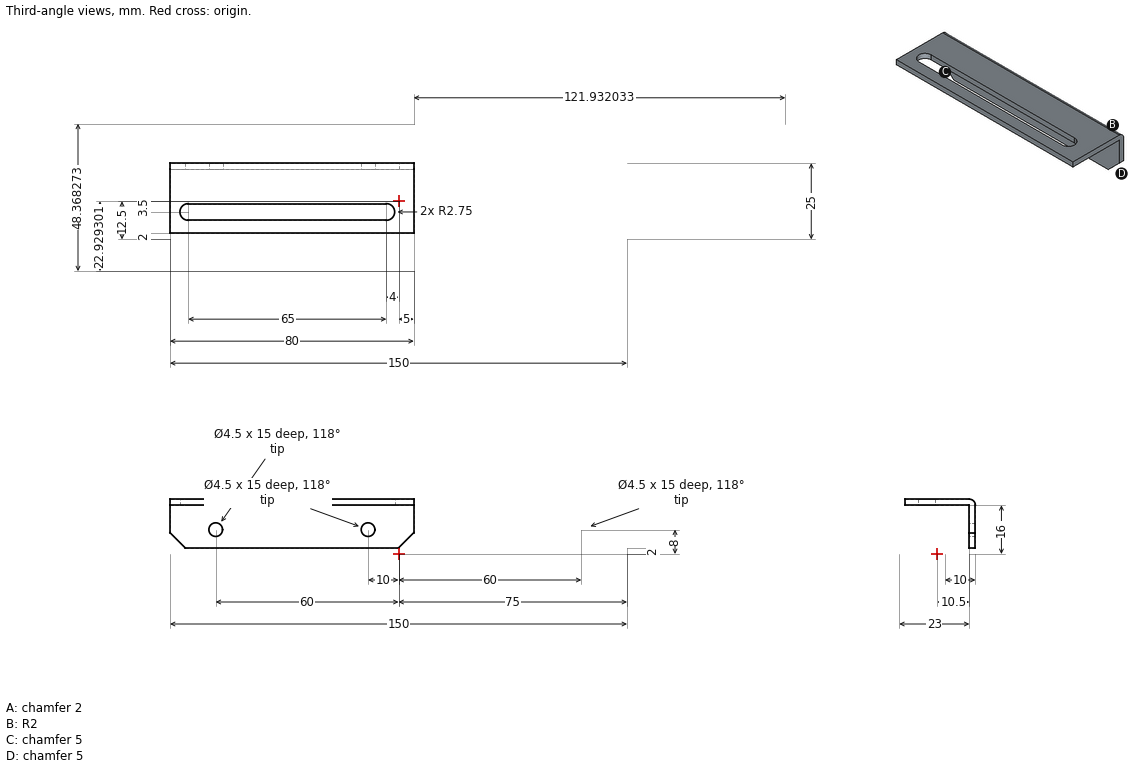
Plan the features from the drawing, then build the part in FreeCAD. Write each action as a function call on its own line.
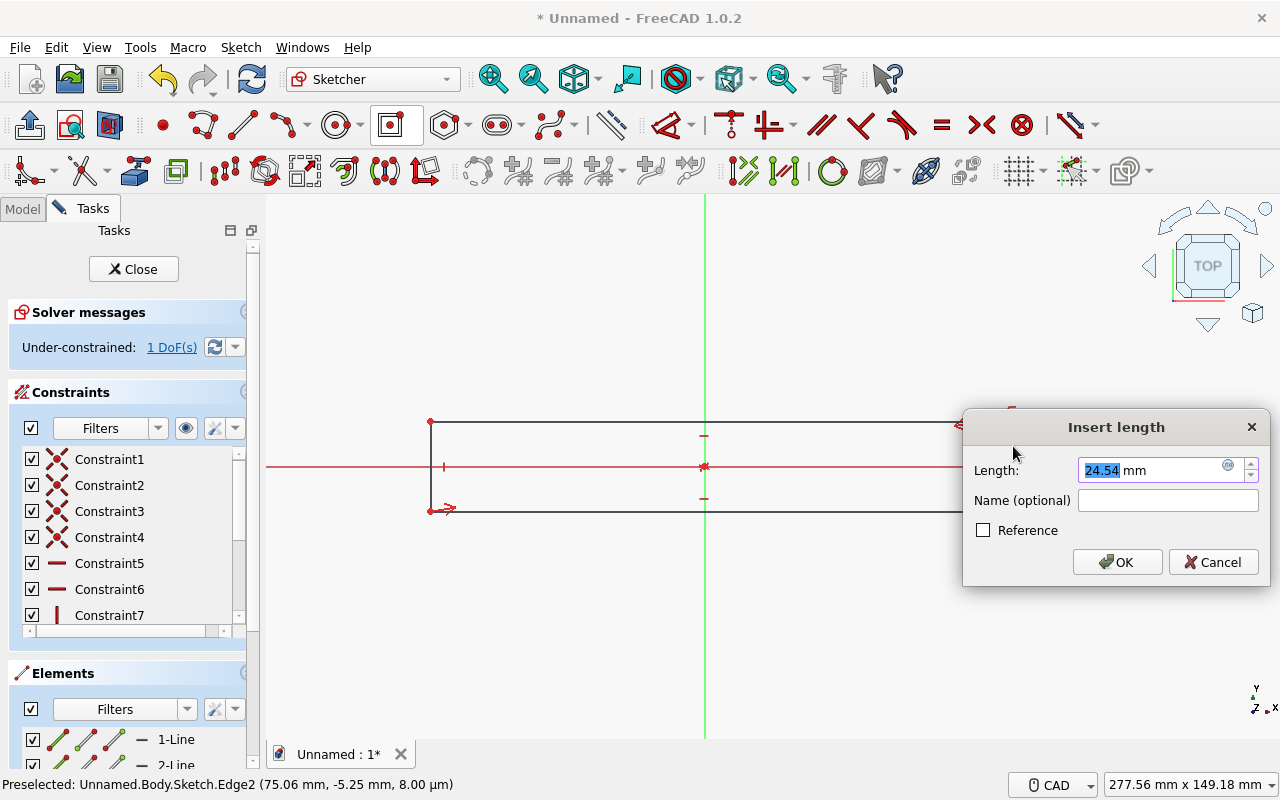
text(25)
key(Return)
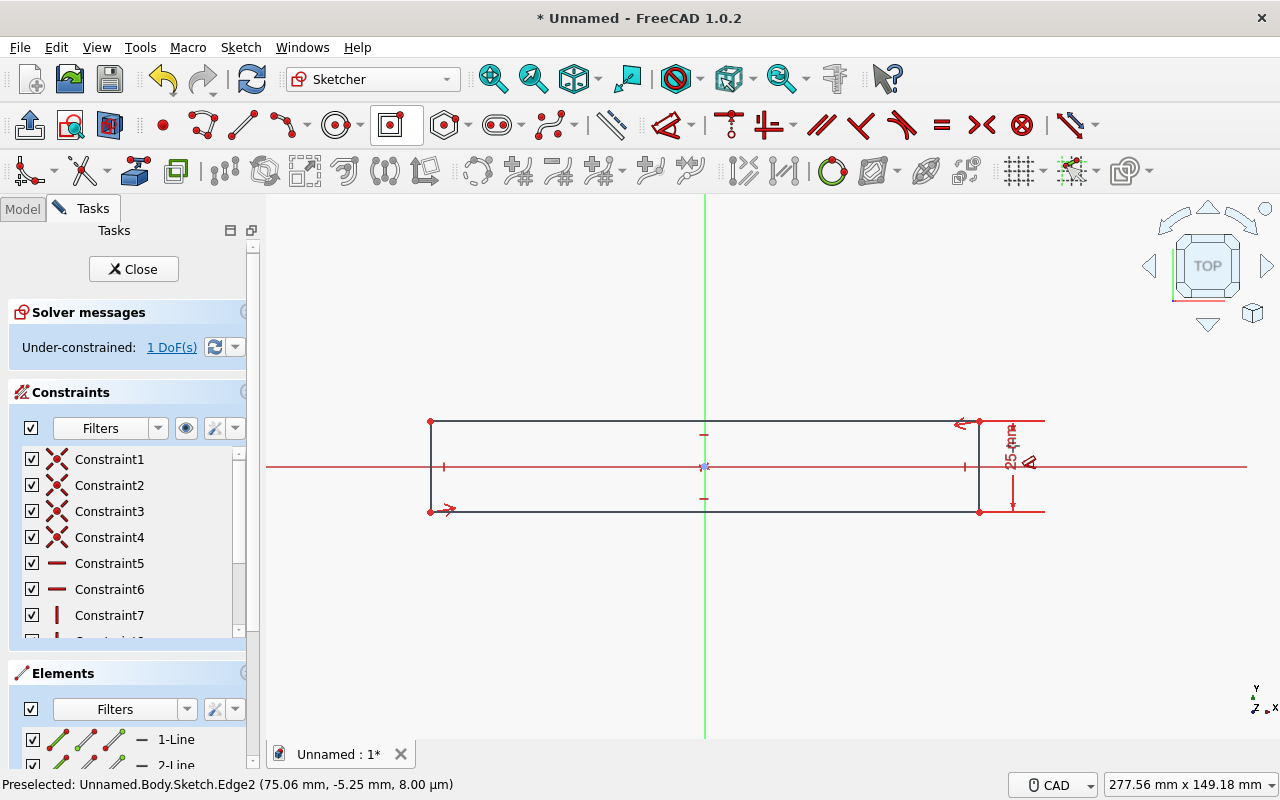
click(595, 512)
click(579, 546)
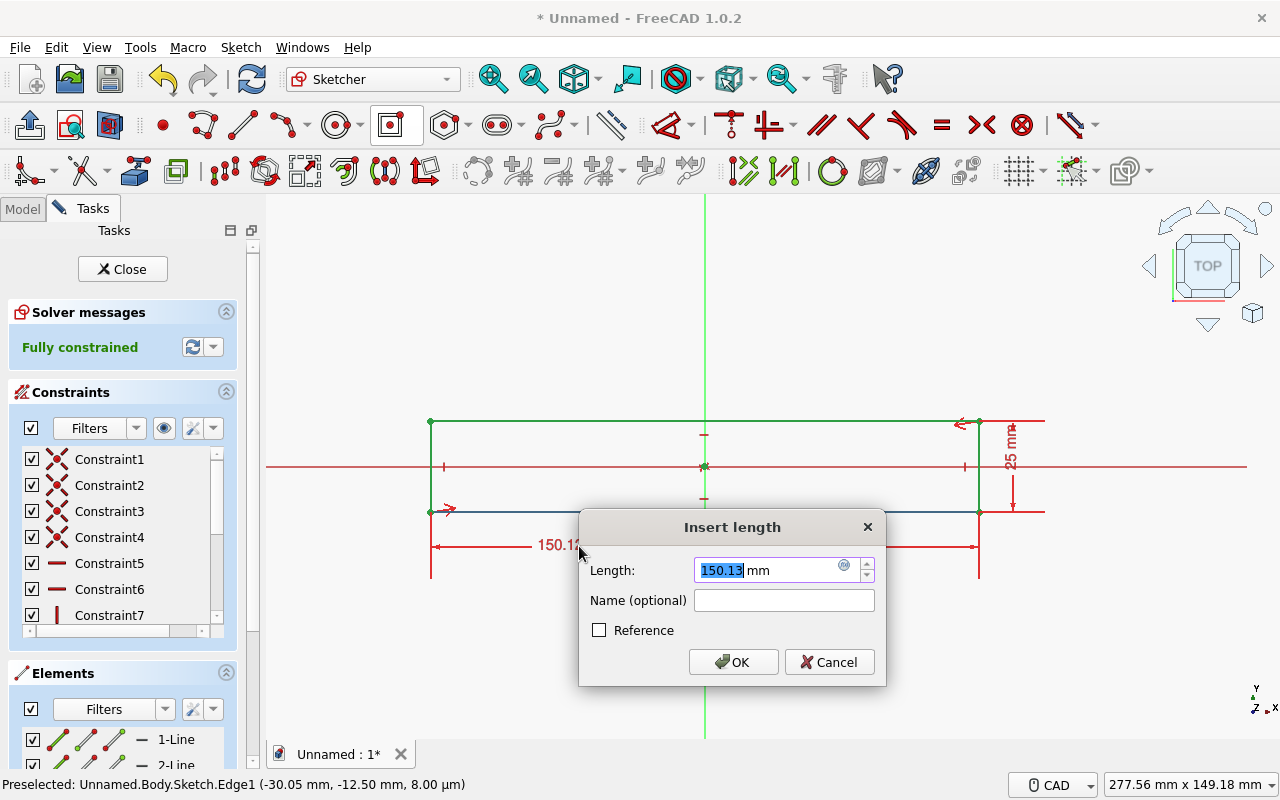
text(150)
key(Return)
key(Escape)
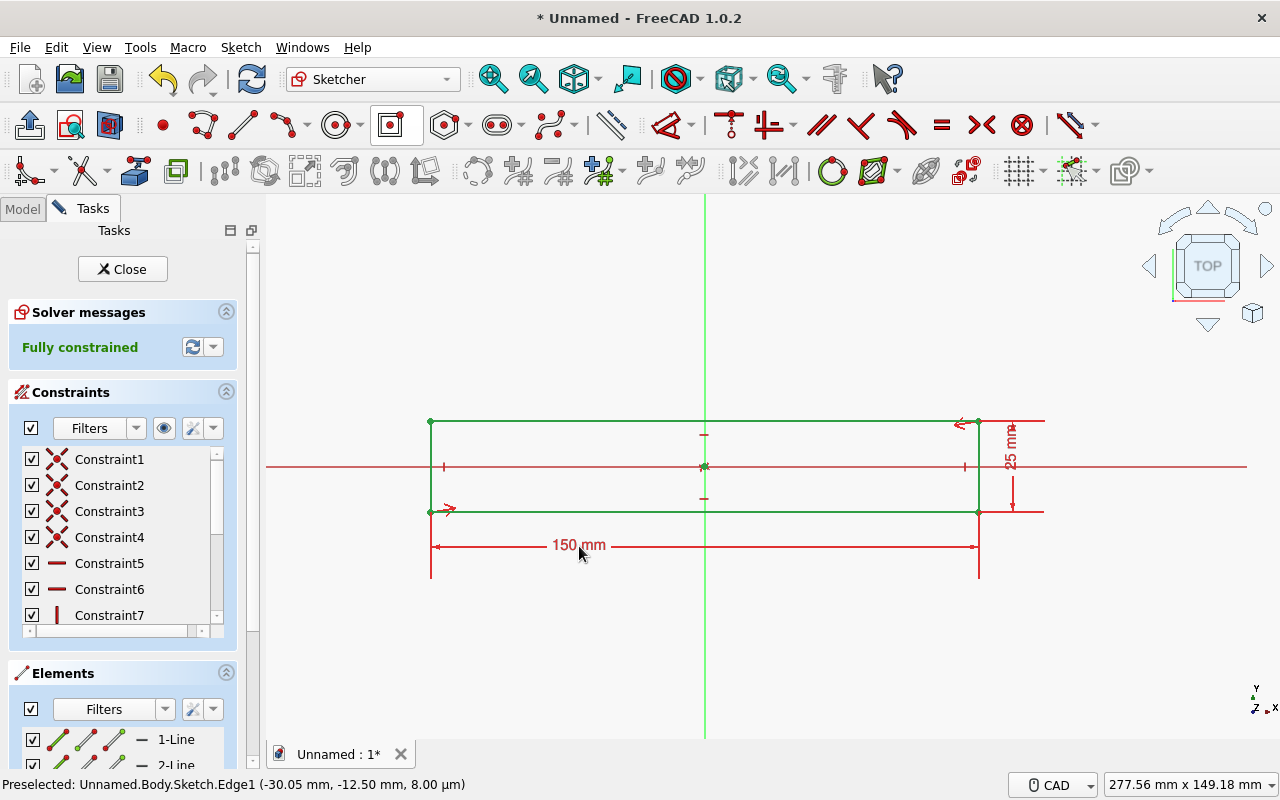
click(123, 269)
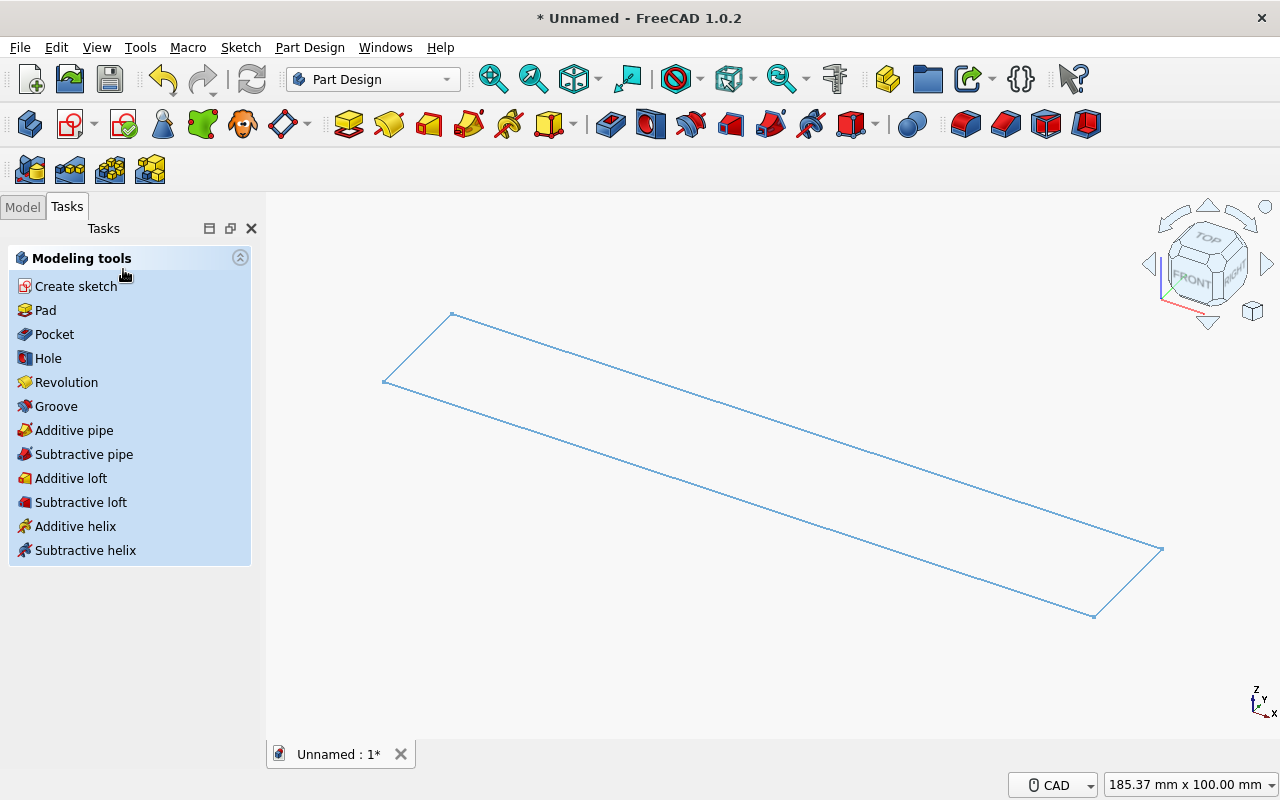
click(350, 124)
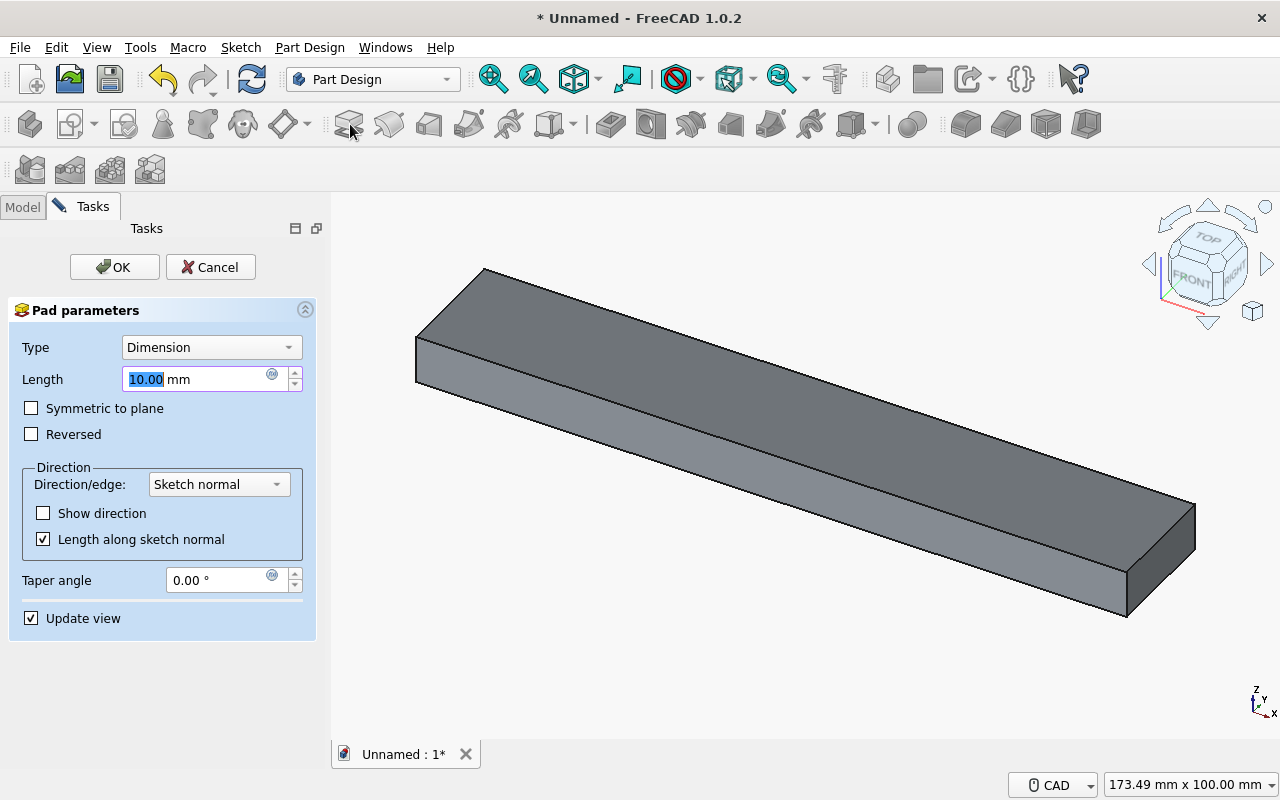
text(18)
key(Tab)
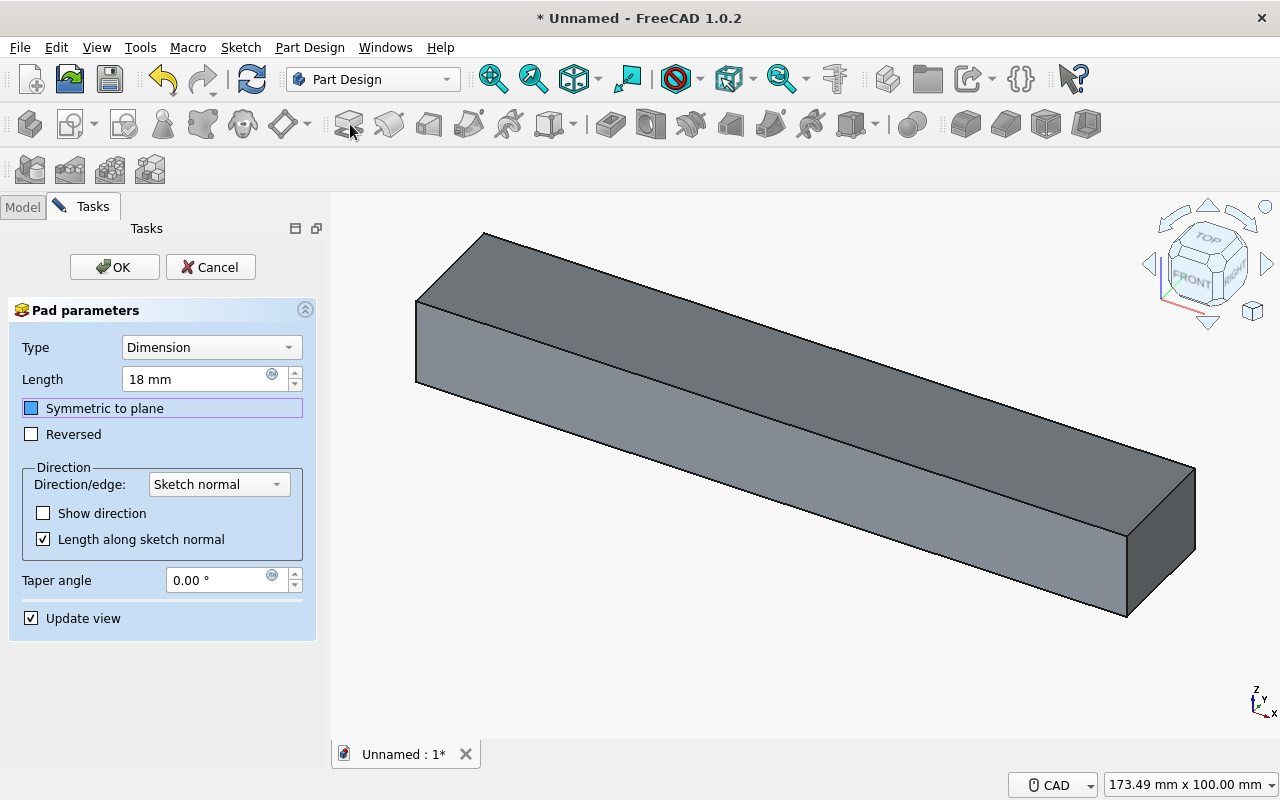
click(115, 267)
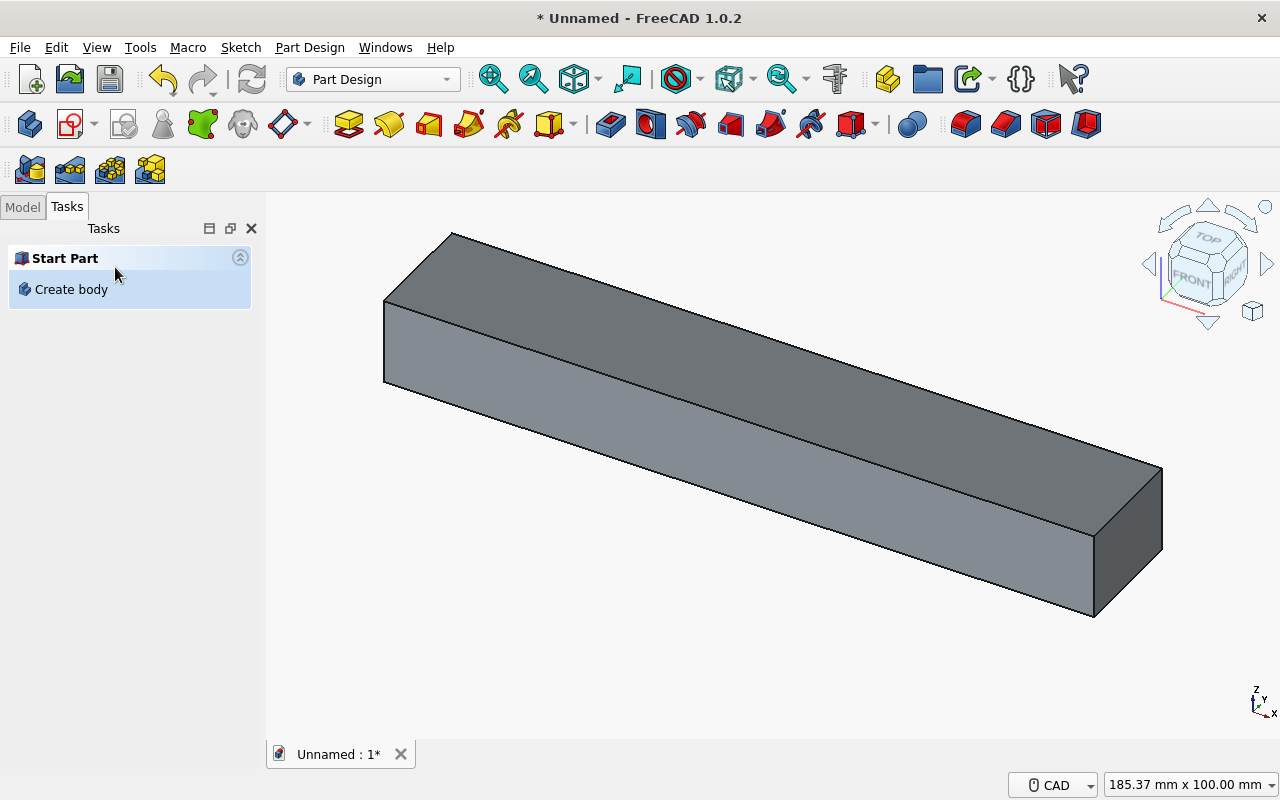
key(6)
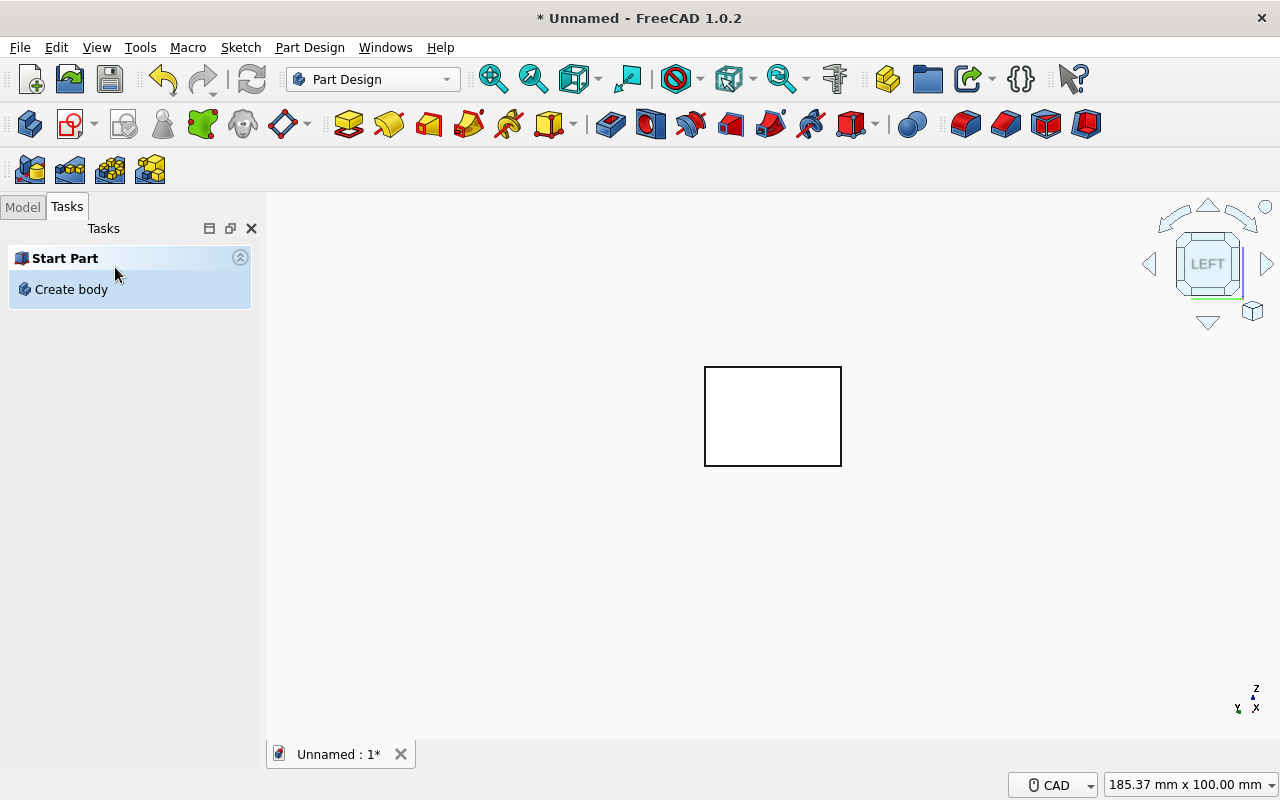
key(v)
key(f)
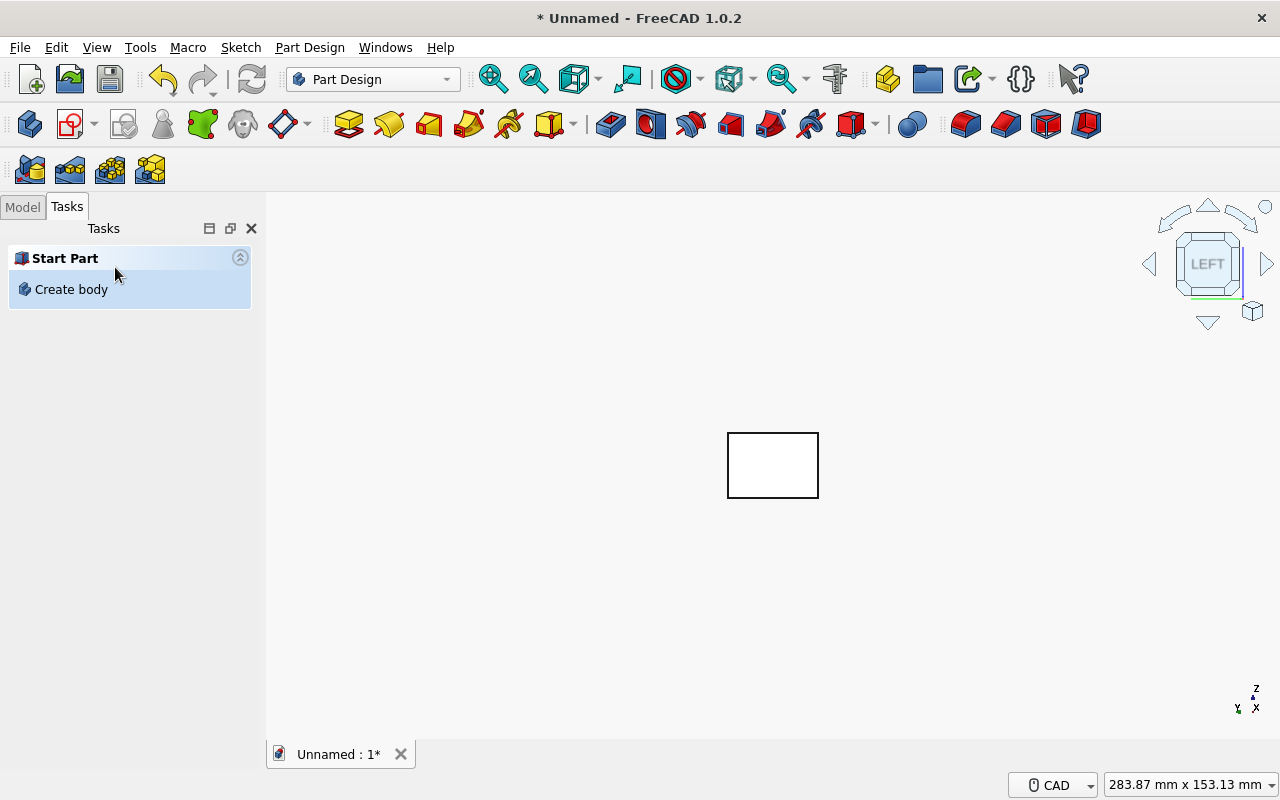
click(773, 464)